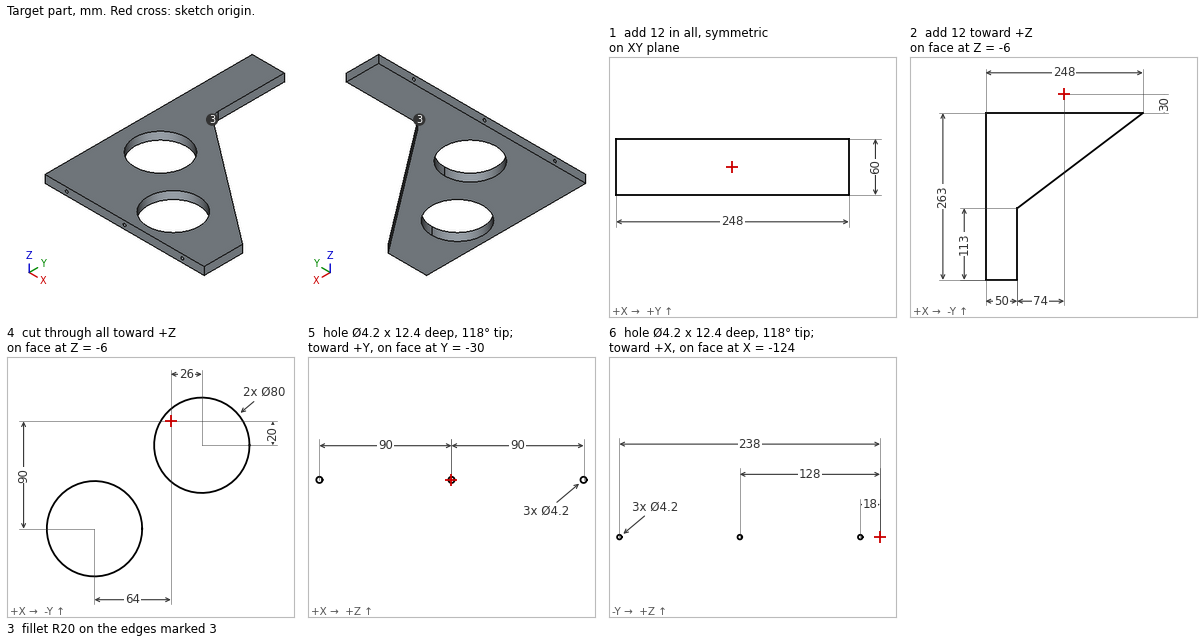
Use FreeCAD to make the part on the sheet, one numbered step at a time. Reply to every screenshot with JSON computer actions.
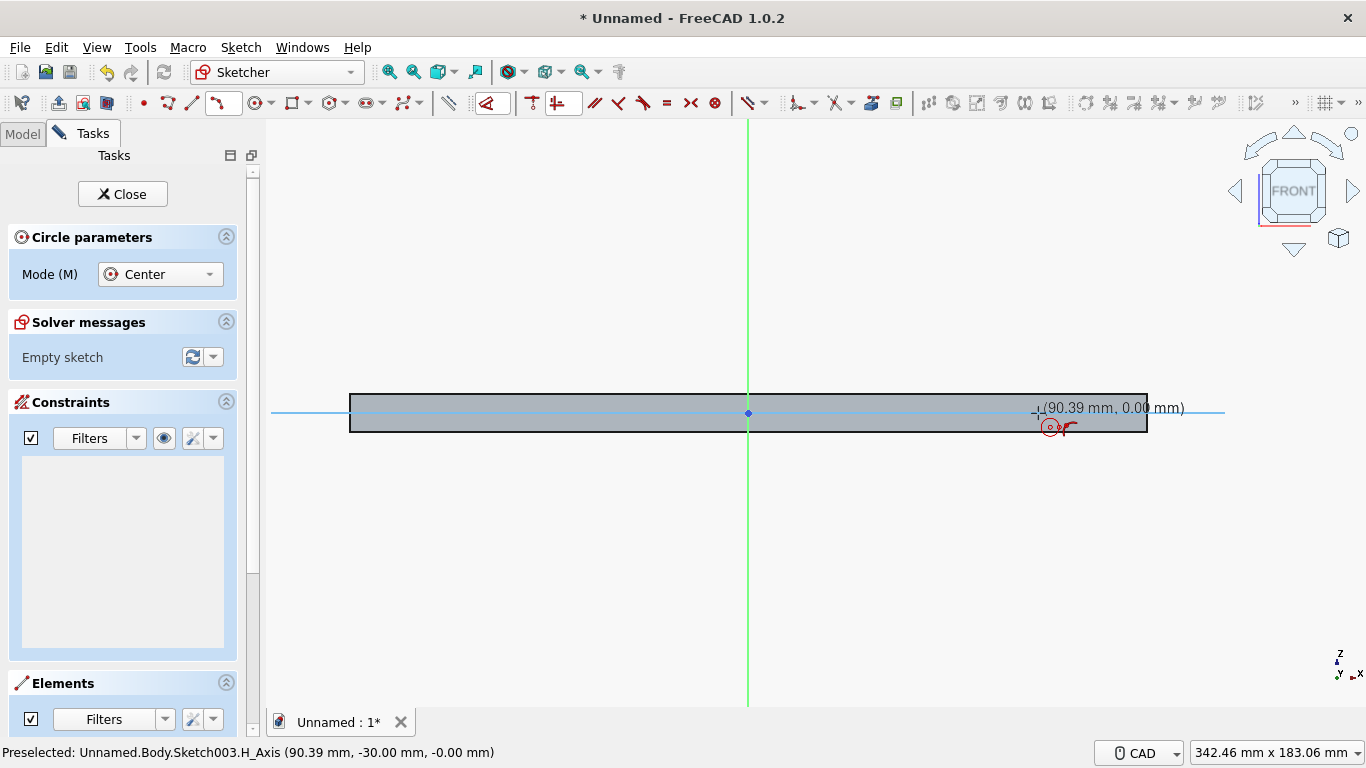
{"action": "left_click", "coordinate": [1037, 413]}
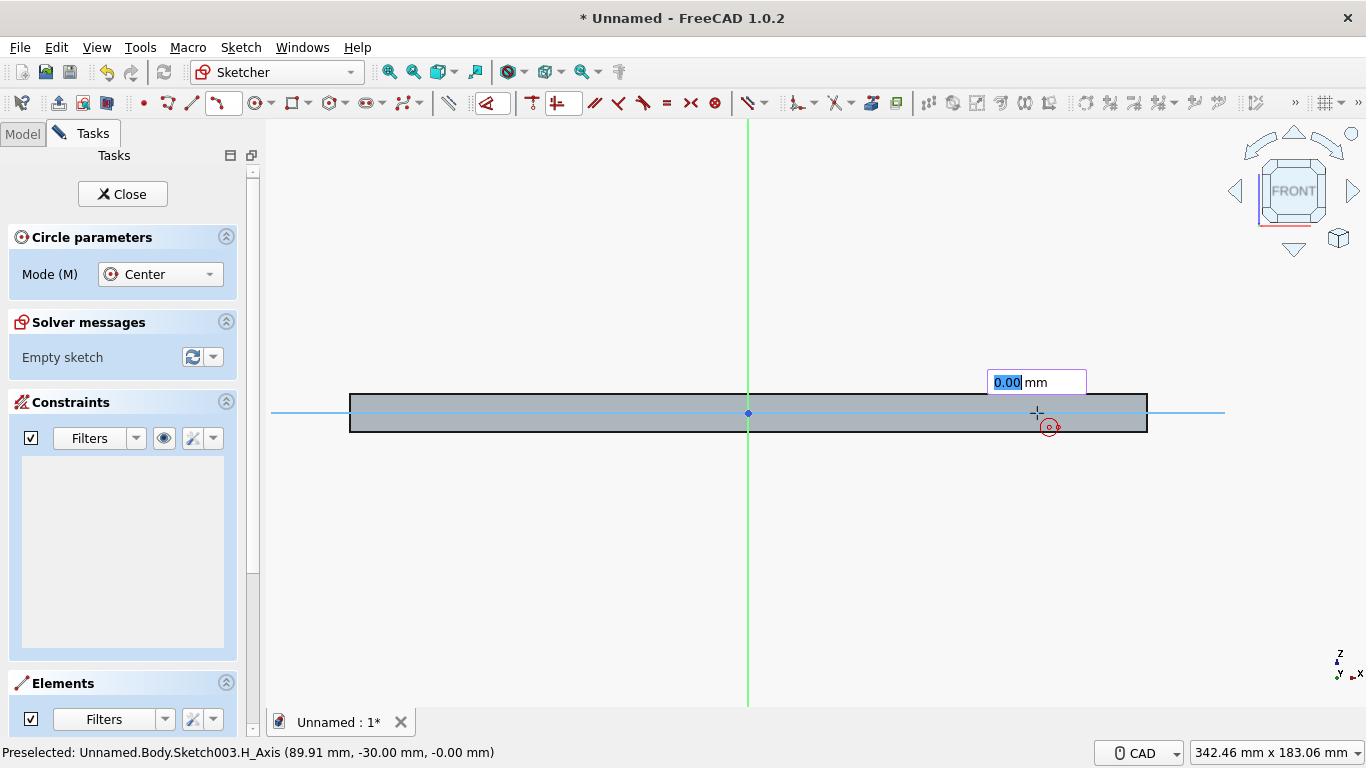
{"action": "scroll", "coordinate": [1035, 419], "scroll_direction": "up", "scroll_amount": 5}
{"action": "mouse_move", "coordinate": [1034, 419]}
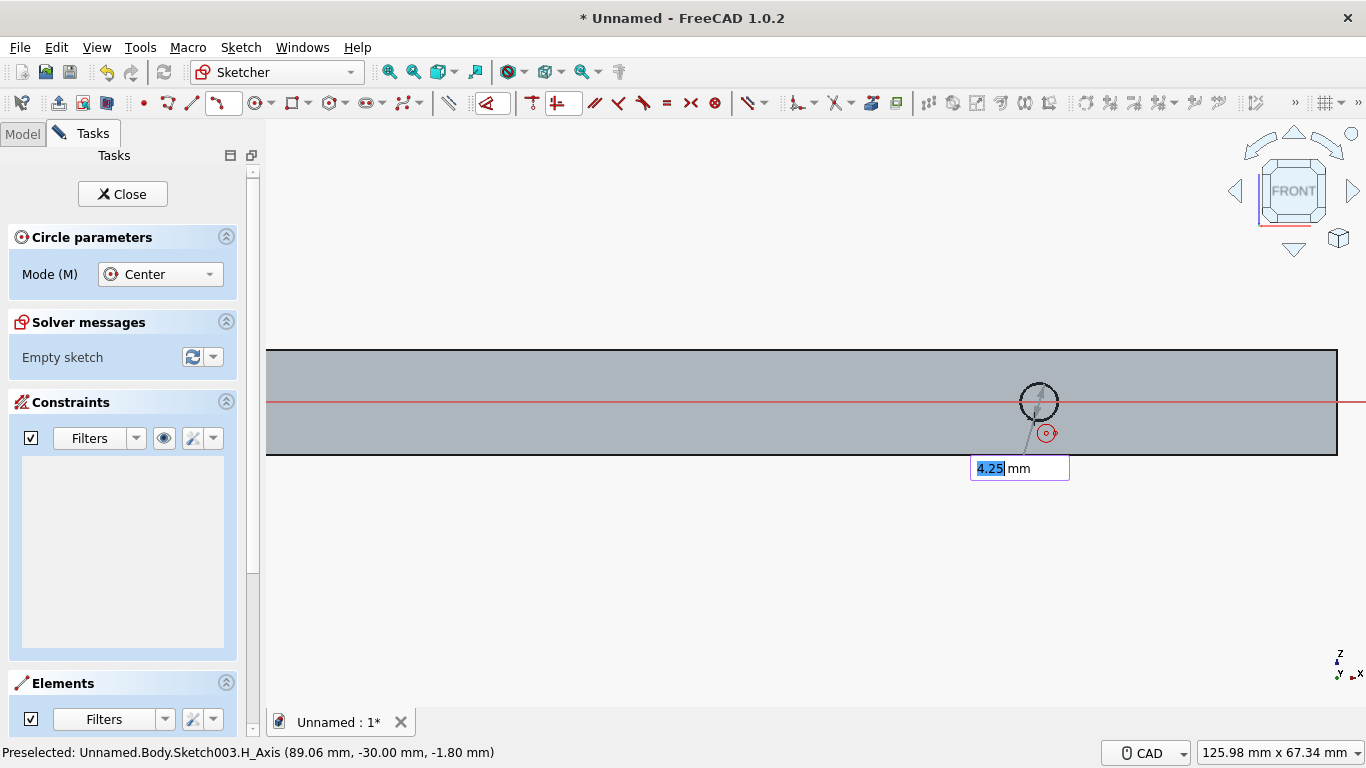
{"action": "type", "text": "4.2"}
{"action": "key", "text": "Return"}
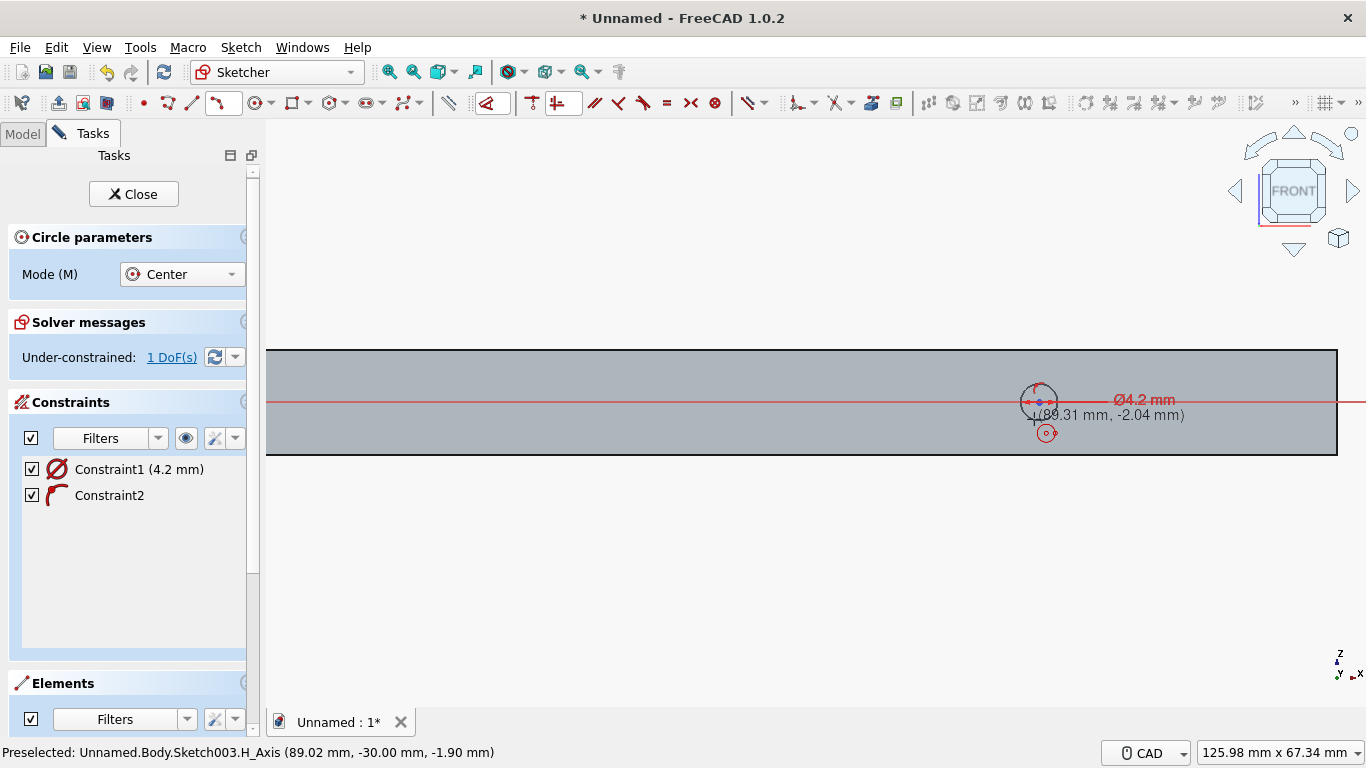
{"action": "scroll", "coordinate": [1035, 419], "scroll_direction": "down", "scroll_amount": 5}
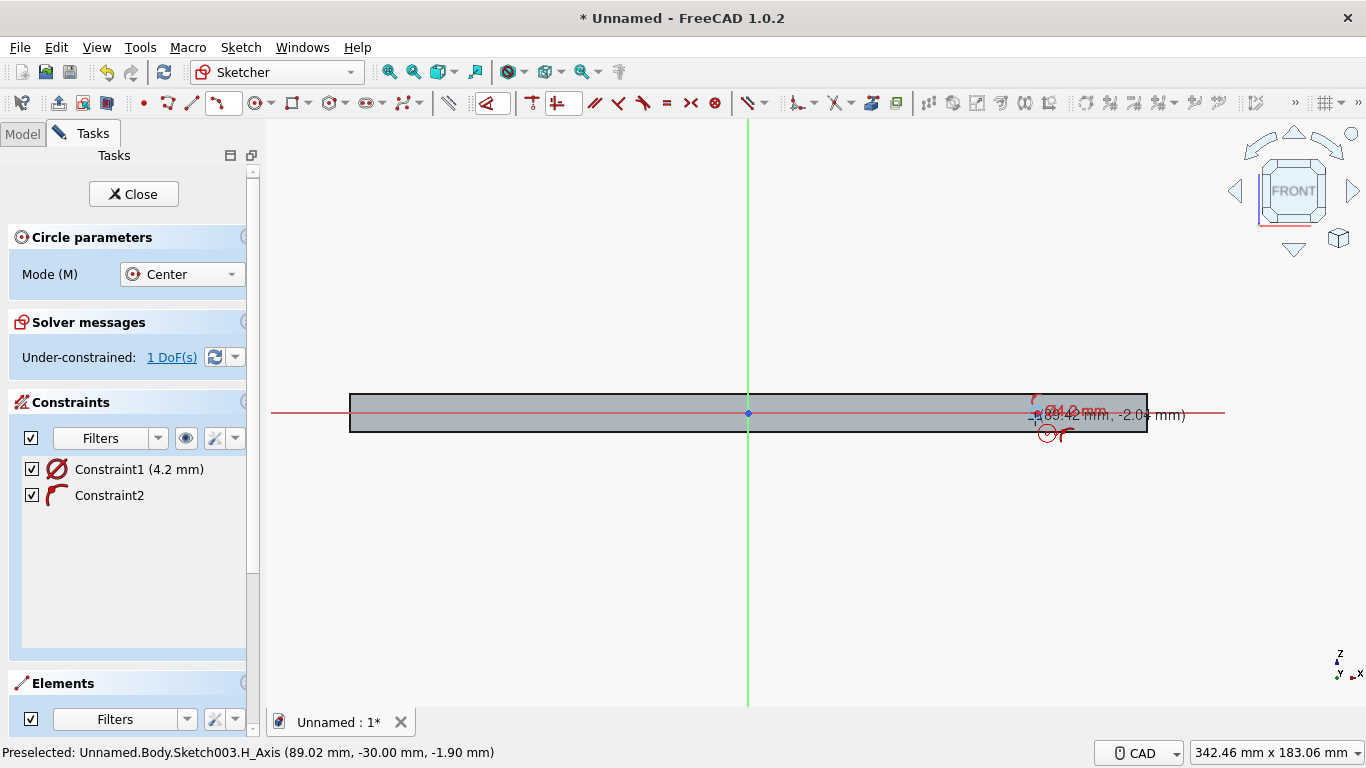
{"action": "scroll", "coordinate": [748, 413], "scroll_direction": "up", "scroll_amount": 7}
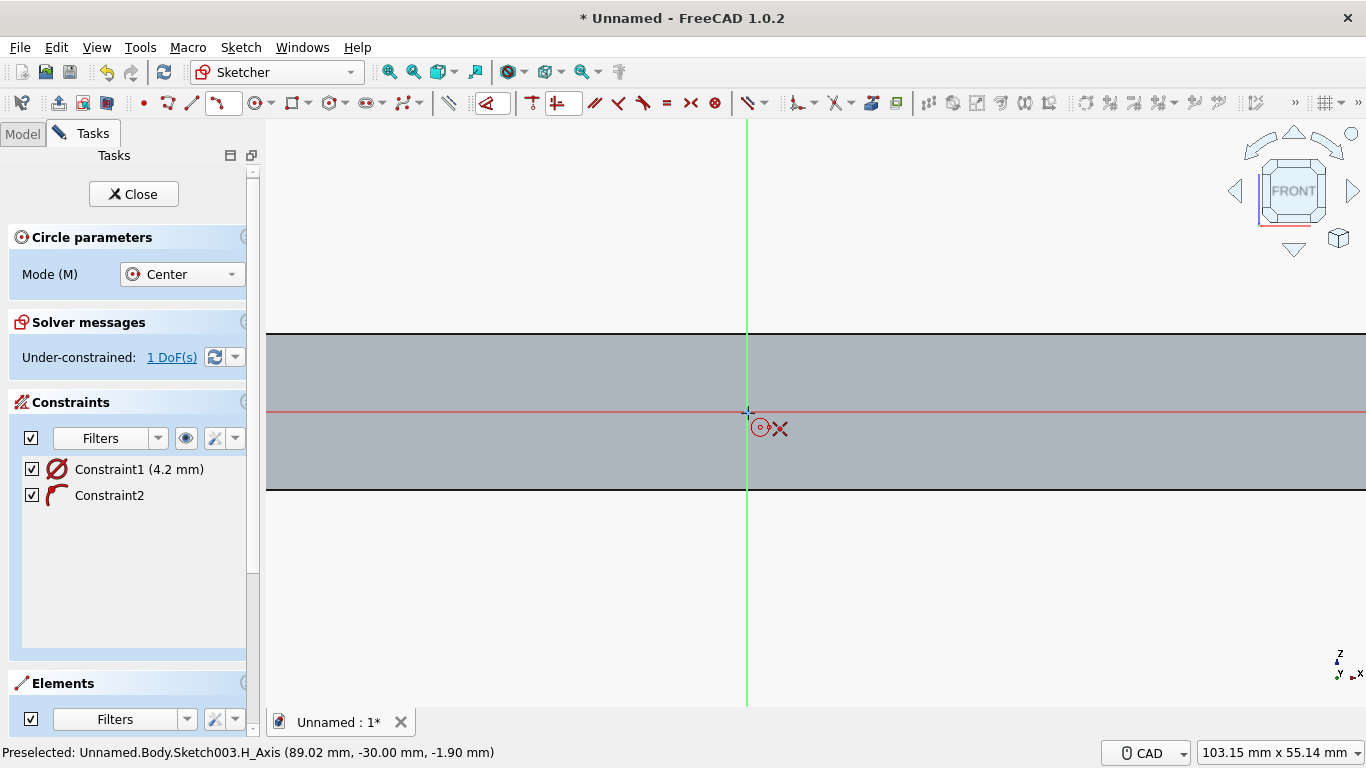
{"action": "scroll", "coordinate": [748, 413], "scroll_direction": "down", "scroll_amount": 7}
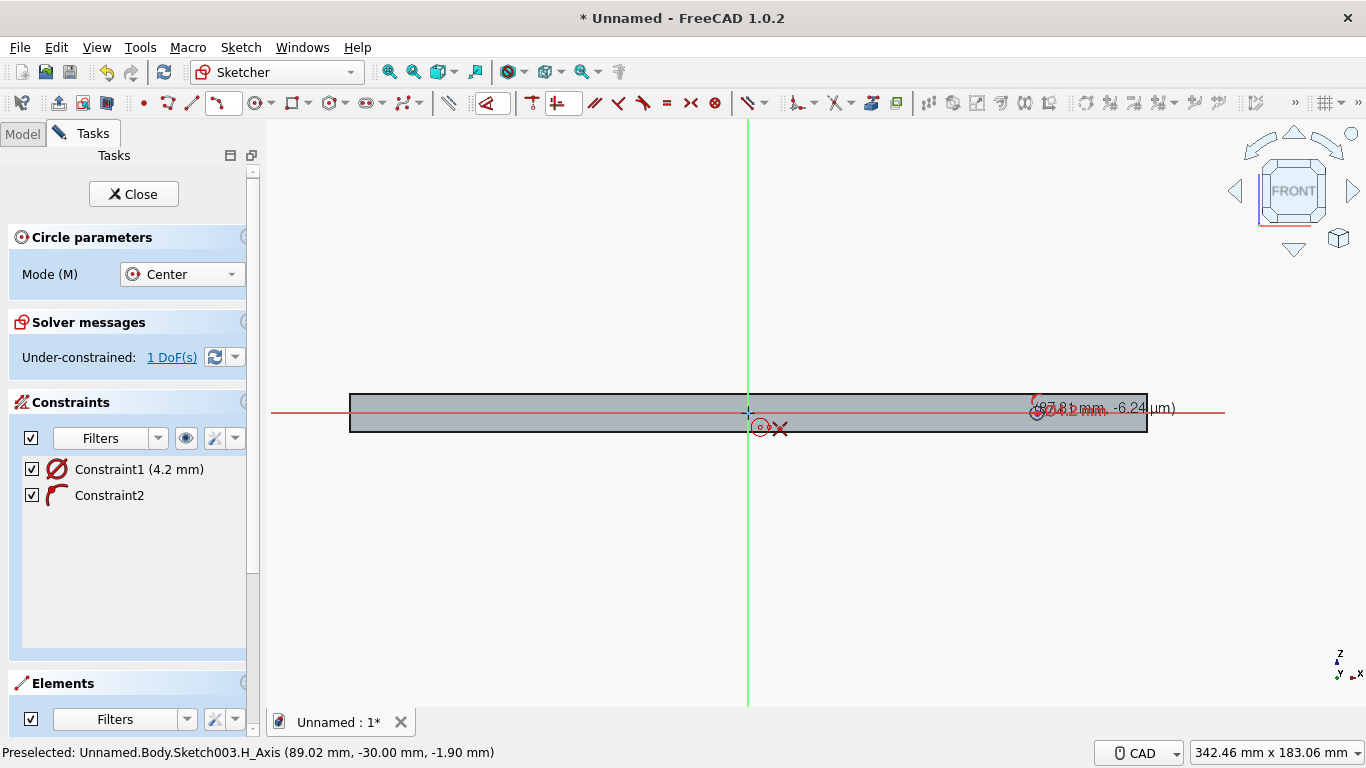
{"action": "left_click", "coordinate": [748, 413]}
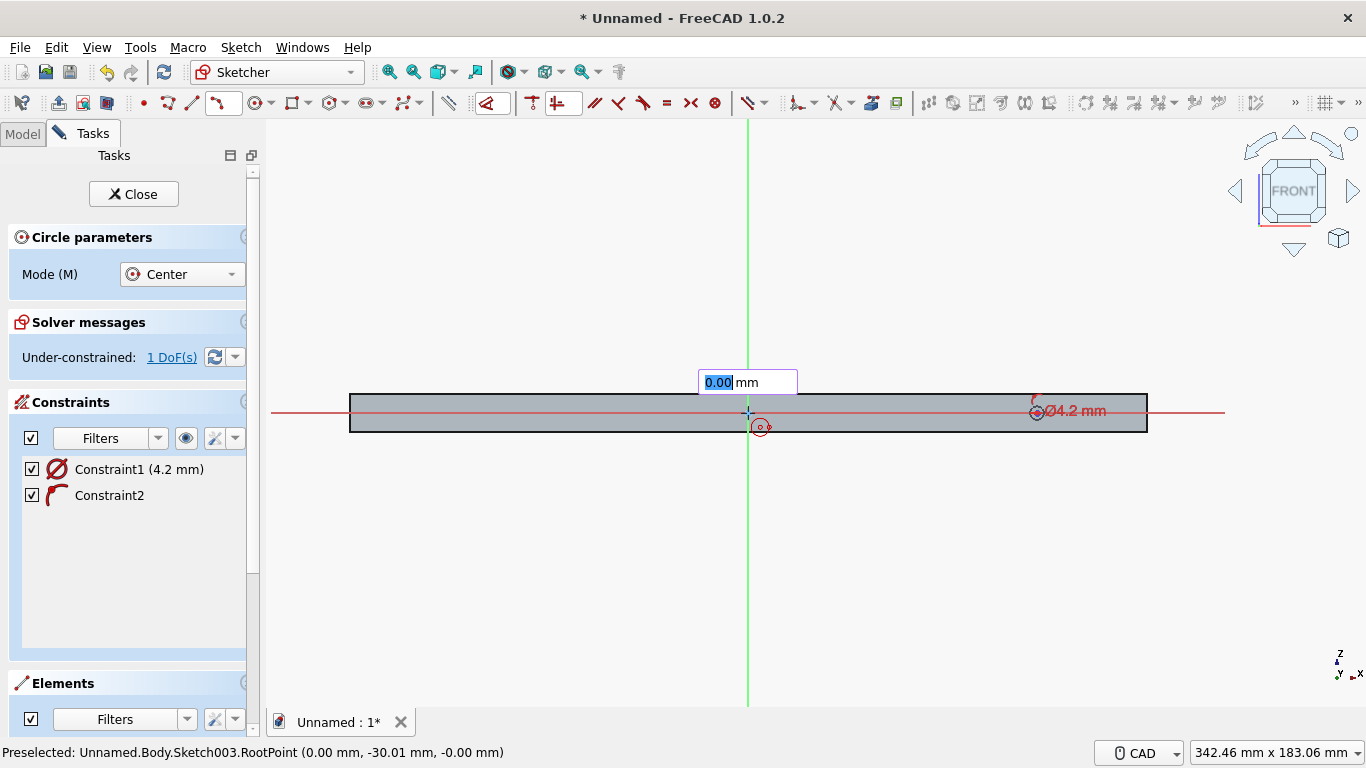
{"action": "scroll", "coordinate": [753, 408], "scroll_direction": "up", "scroll_amount": 7}
{"action": "mouse_move", "coordinate": [752, 408]}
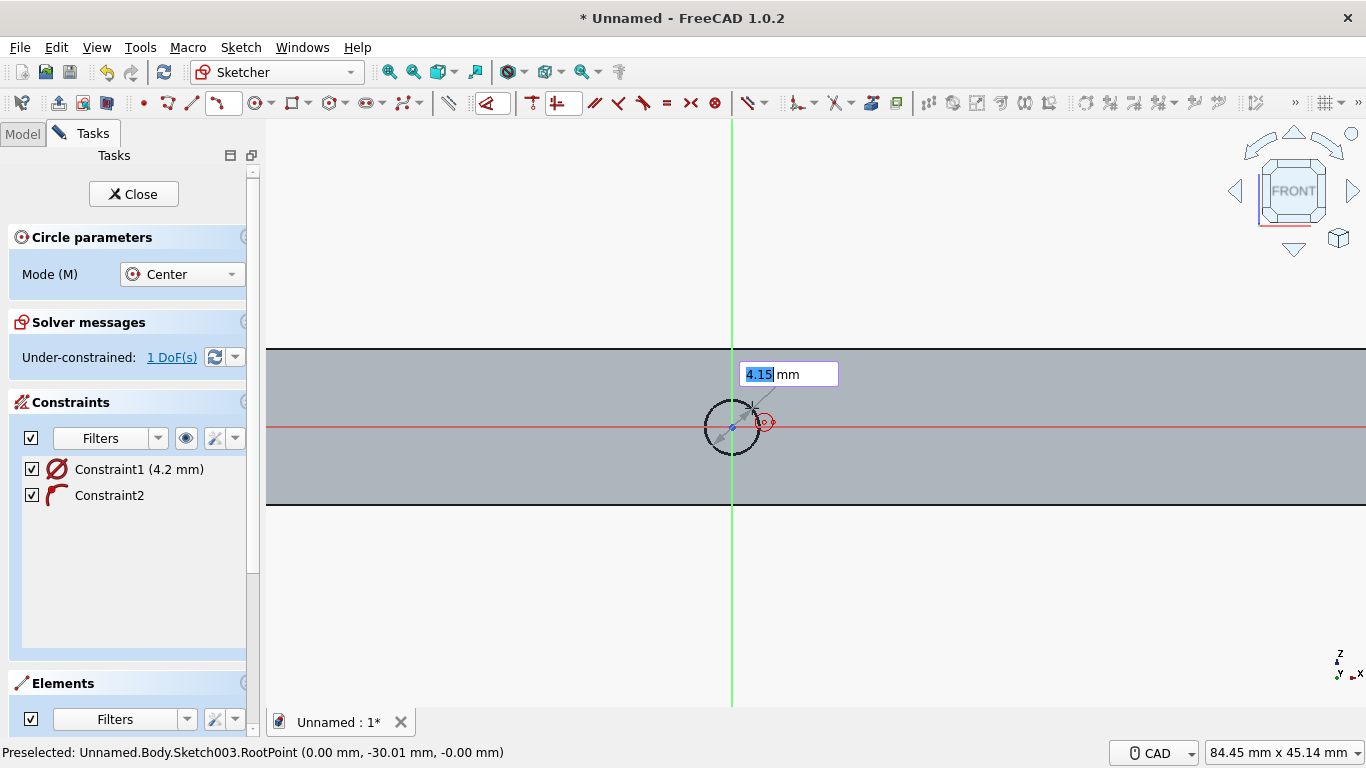
{"action": "type", "text": "4.2"}
{"action": "key", "text": "Return"}